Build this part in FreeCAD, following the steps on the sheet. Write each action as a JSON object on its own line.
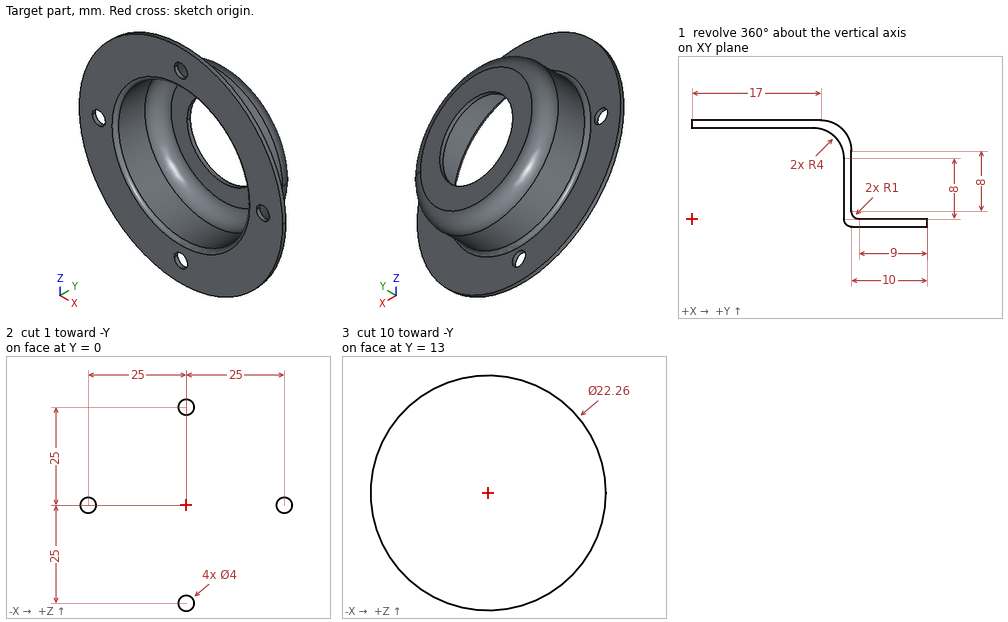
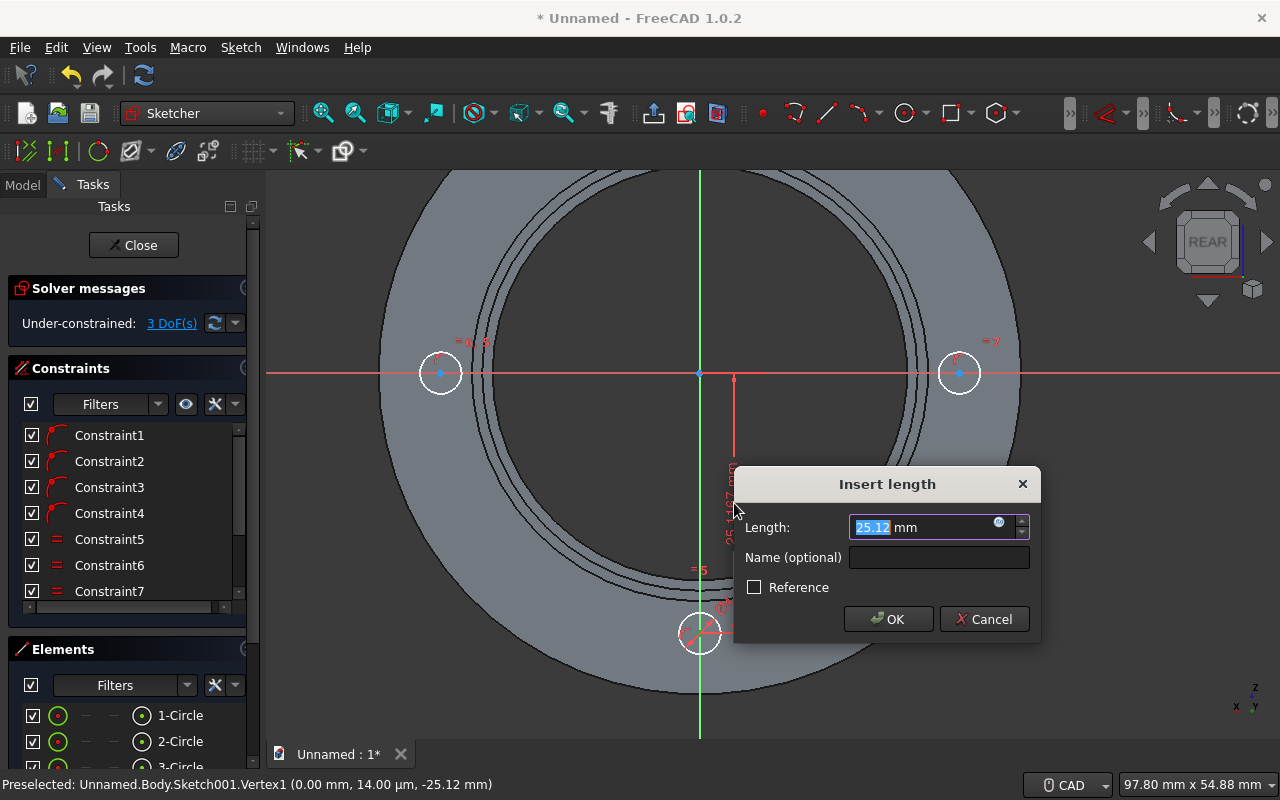
{"action": "type", "text": "25"}
{"action": "key", "text": "Return"}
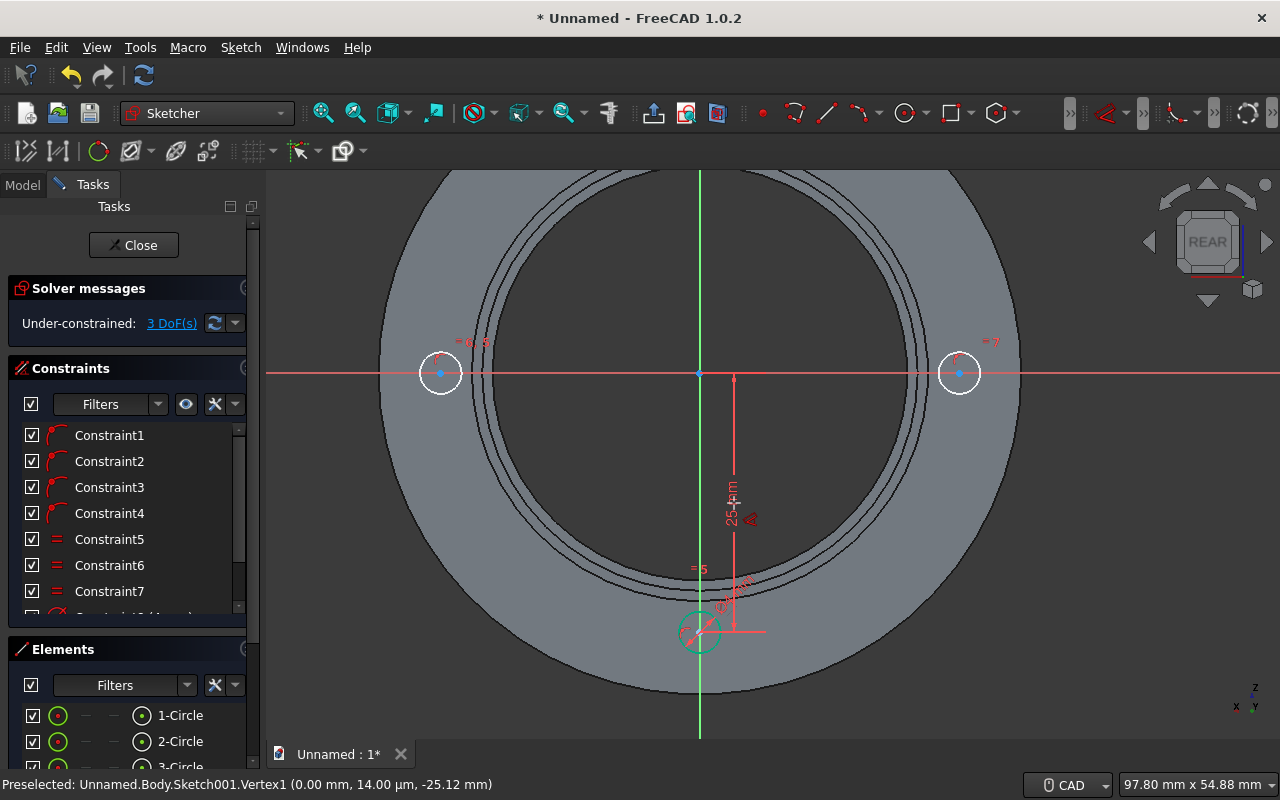
{"action": "left_click", "coordinate": [441, 373]}
{"action": "left_click", "coordinate": [570, 407]}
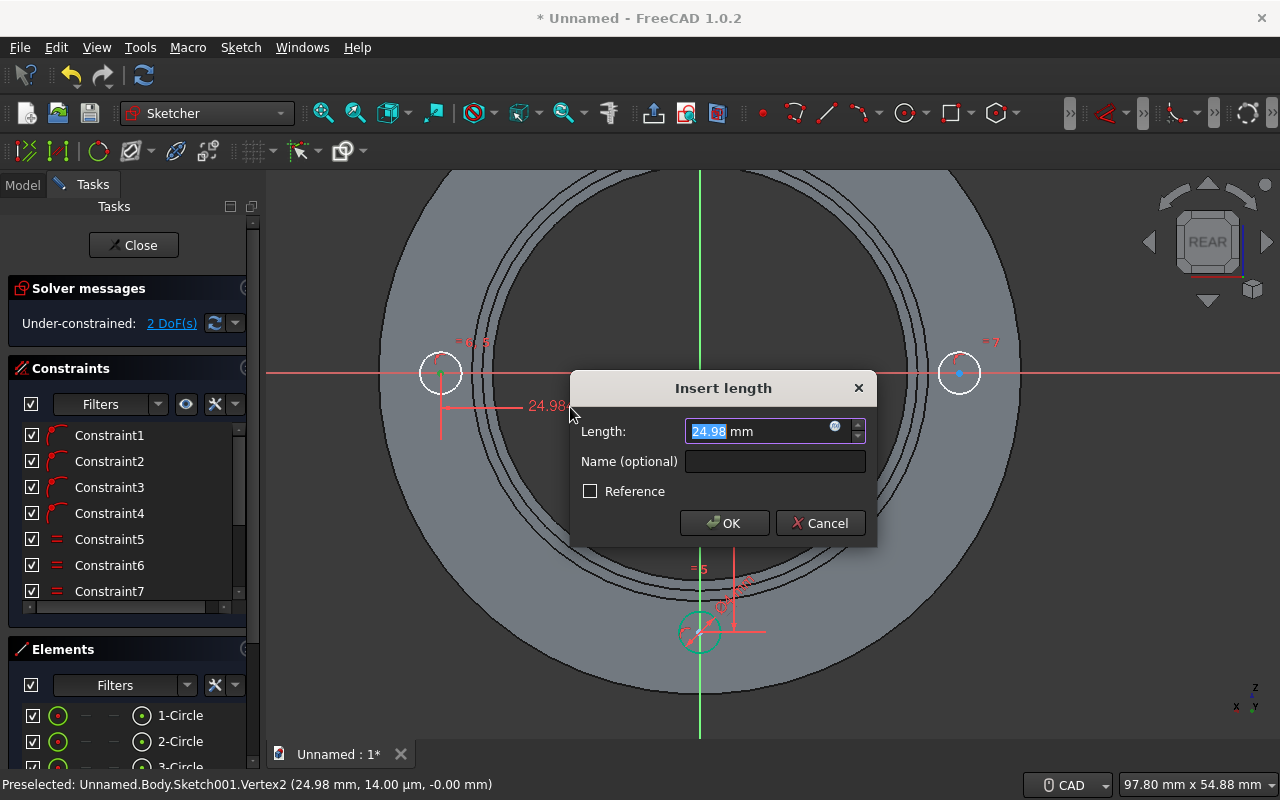
{"action": "type", "text": "25"}
{"action": "key", "text": "Return"}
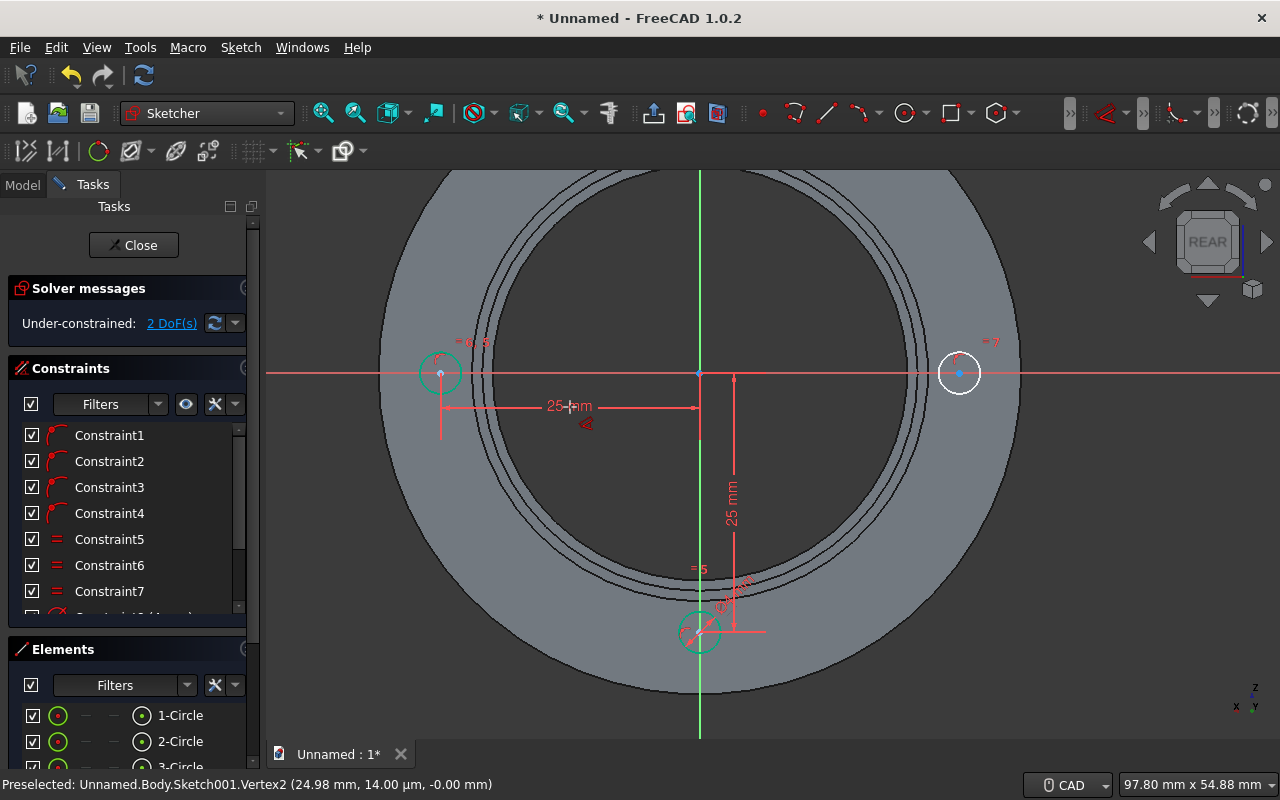
{"action": "scroll", "coordinate": [714, 620], "scroll_direction": "down", "scroll_amount": 2}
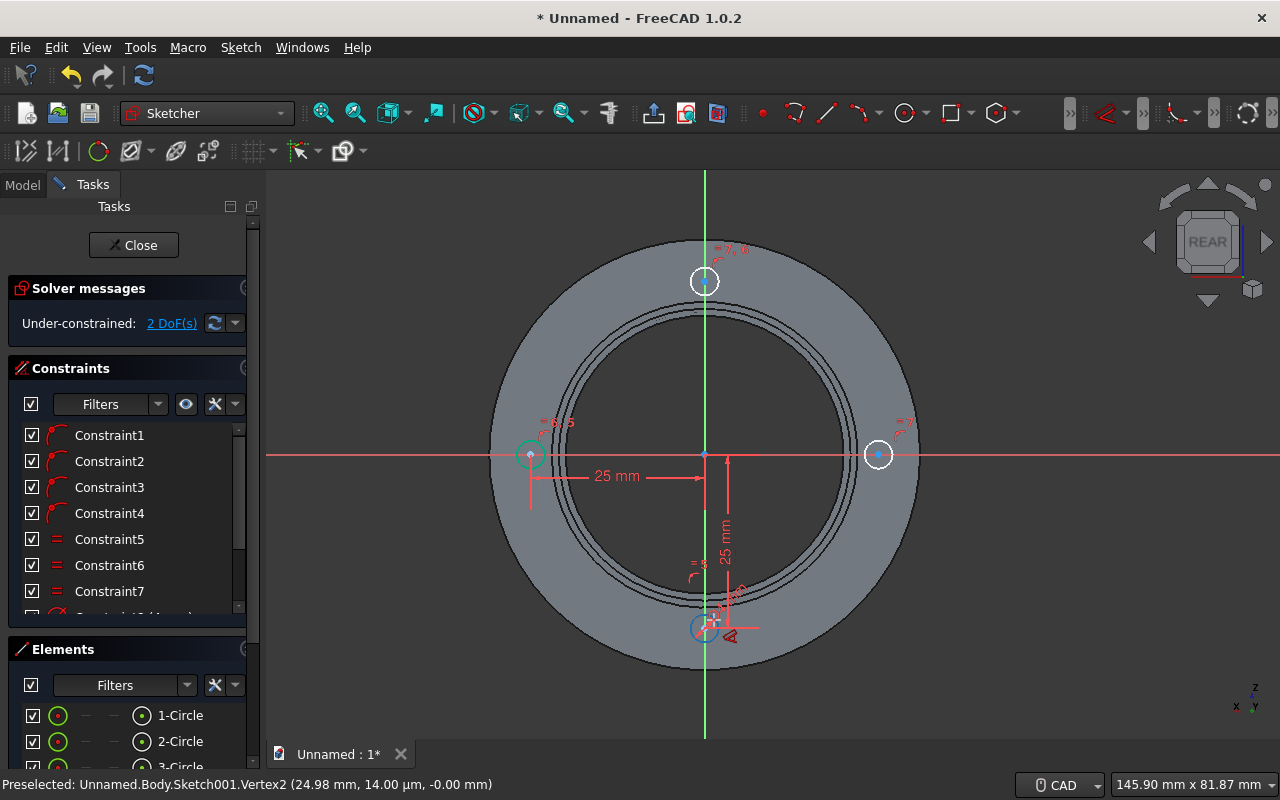
{"action": "left_click", "coordinate": [705, 282]}
{"action": "left_click", "coordinate": [739, 368]}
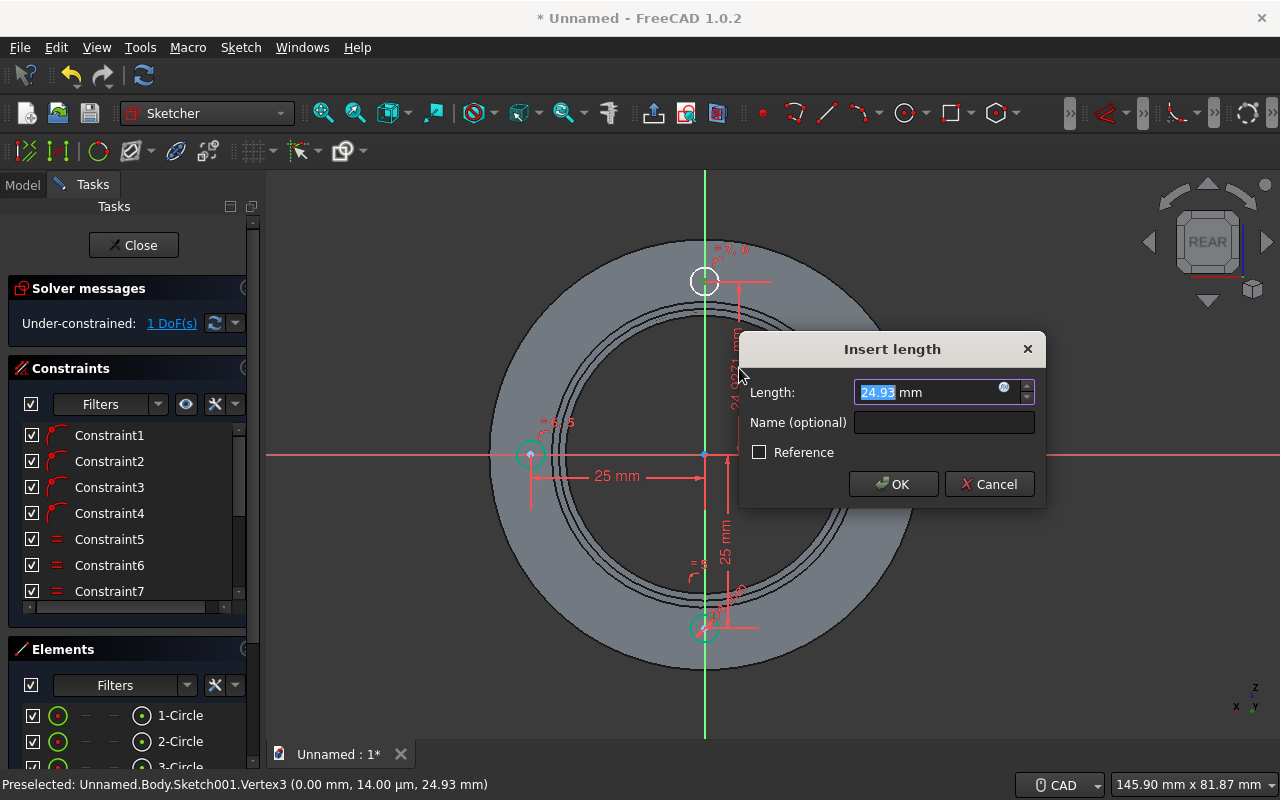
{"action": "type", "text": "25"}
{"action": "key", "text": "Return"}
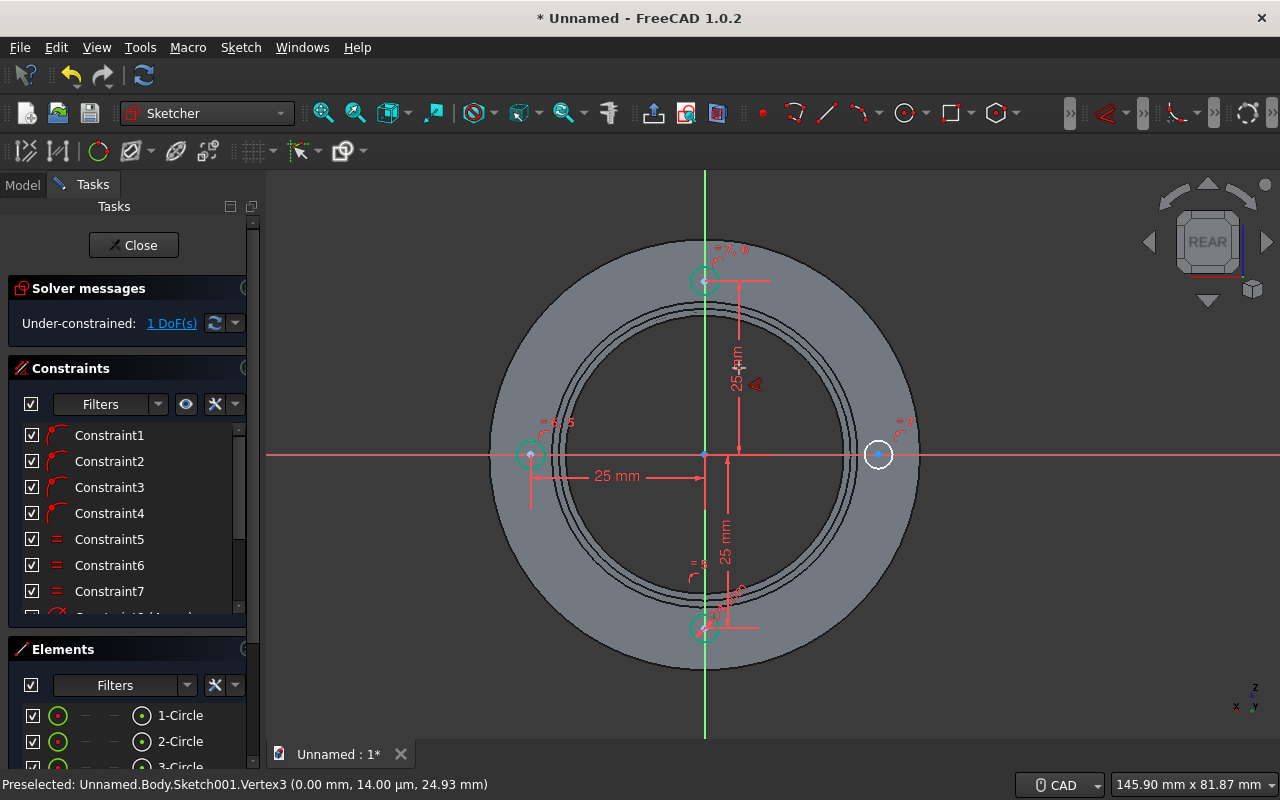
{"action": "left_click", "coordinate": [879, 455]}
{"action": "left_click", "coordinate": [792, 489]}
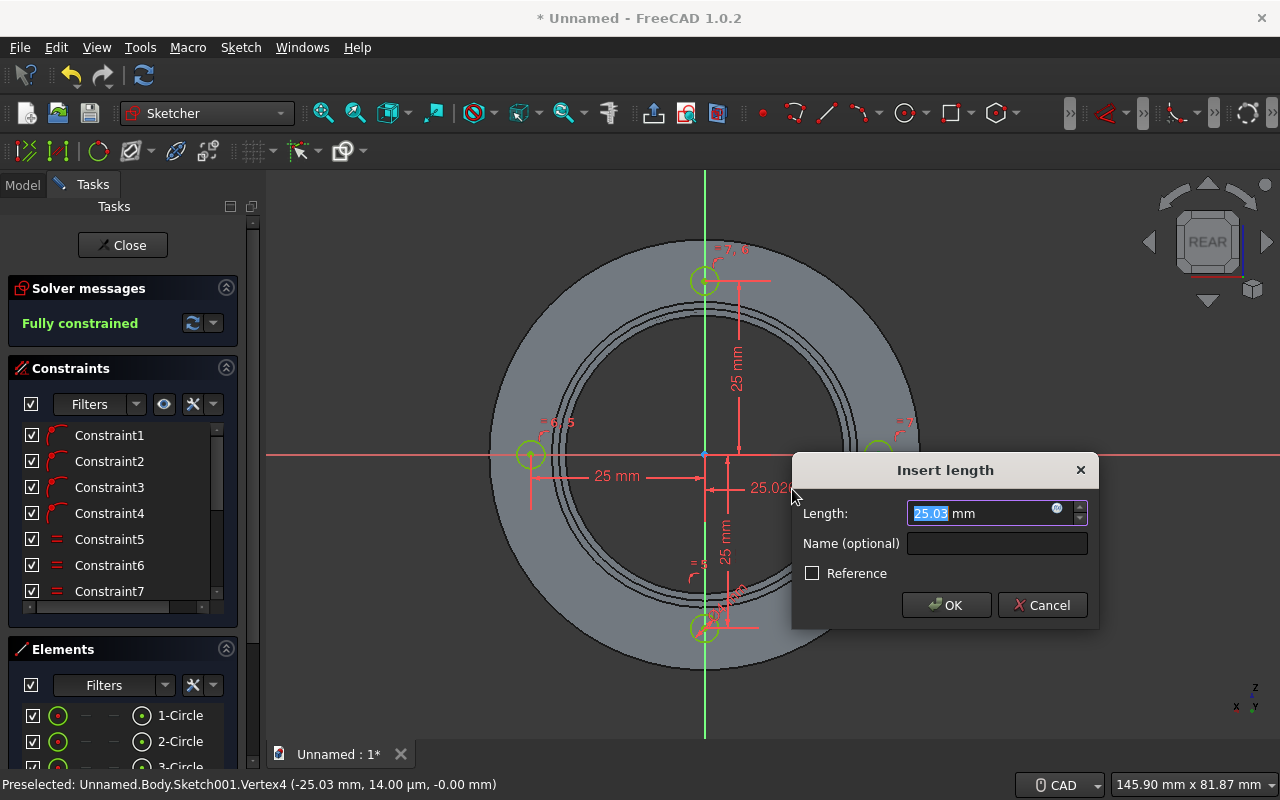
{"action": "type", "text": "25"}
{"action": "key", "text": "Return"}
{"action": "key", "text": "Escape"}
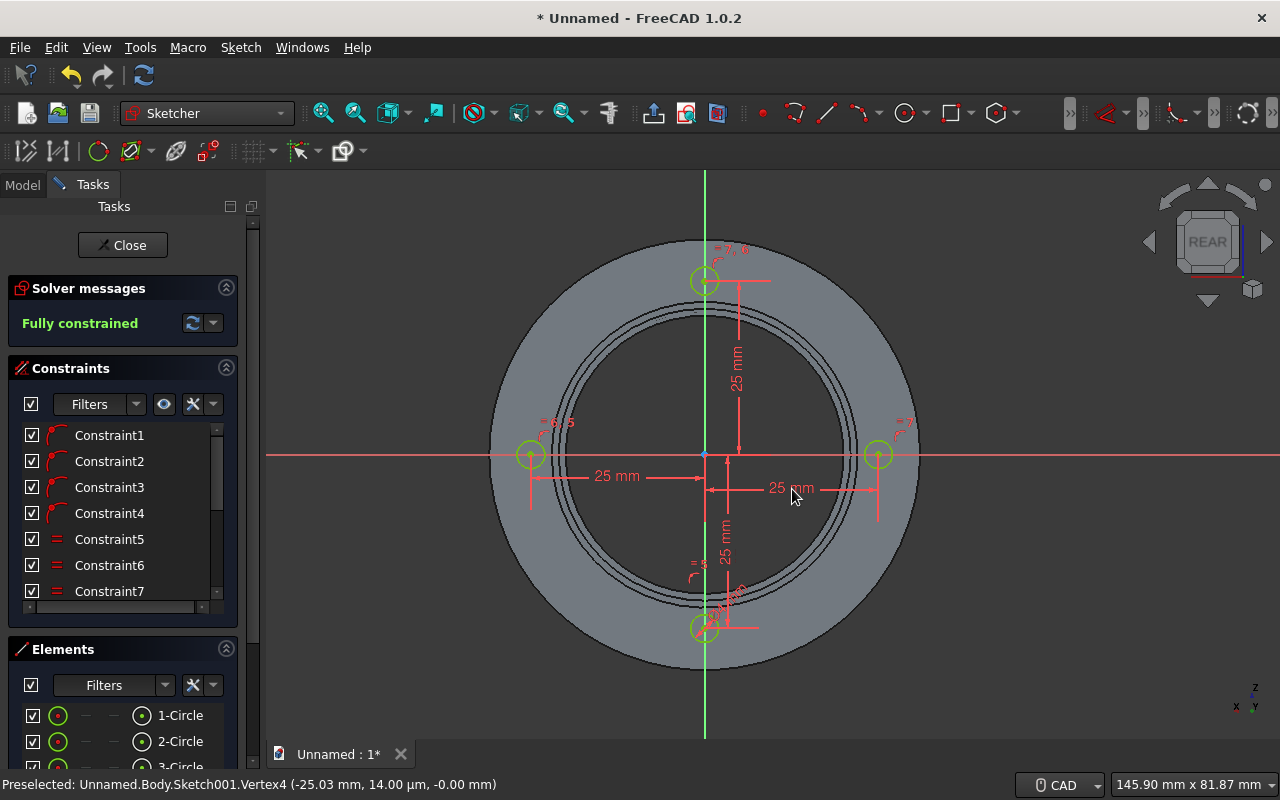
{"action": "left_click", "coordinate": [123, 245]}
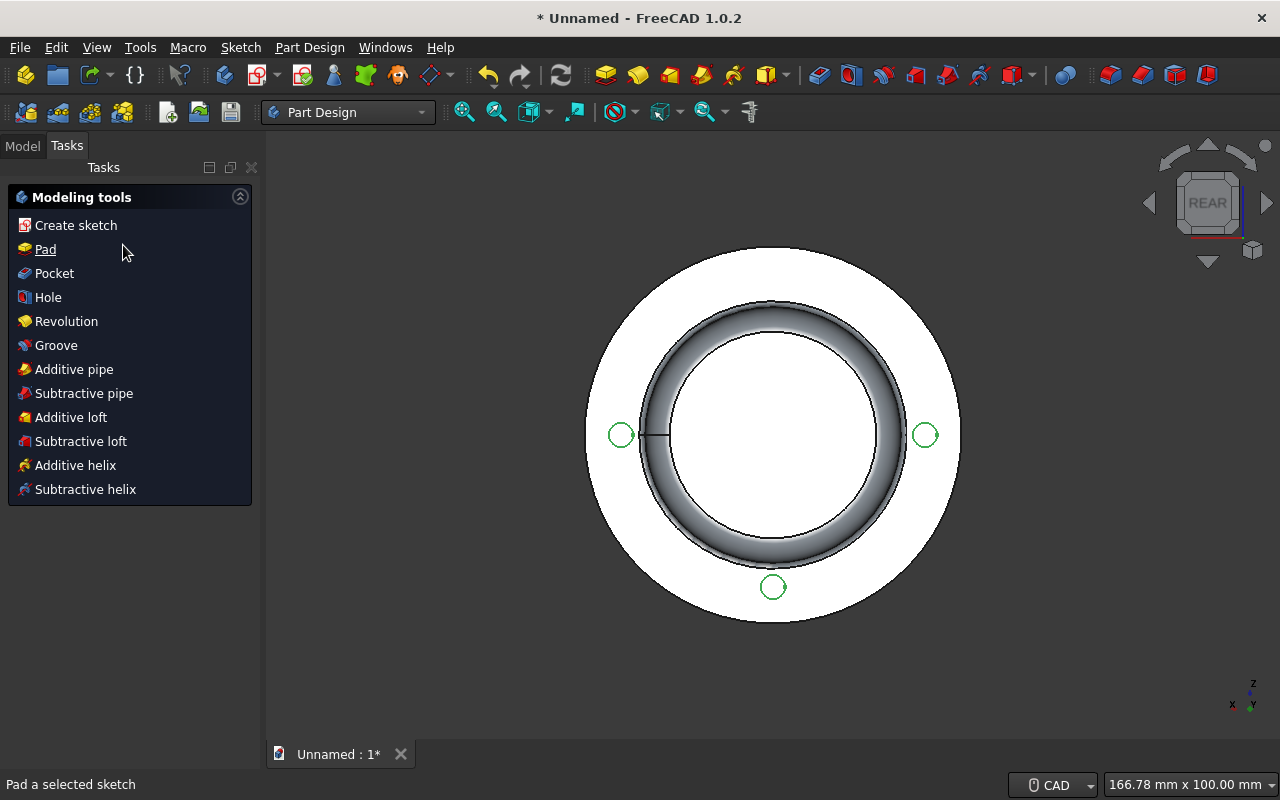
{"action": "left_click", "coordinate": [820, 76]}